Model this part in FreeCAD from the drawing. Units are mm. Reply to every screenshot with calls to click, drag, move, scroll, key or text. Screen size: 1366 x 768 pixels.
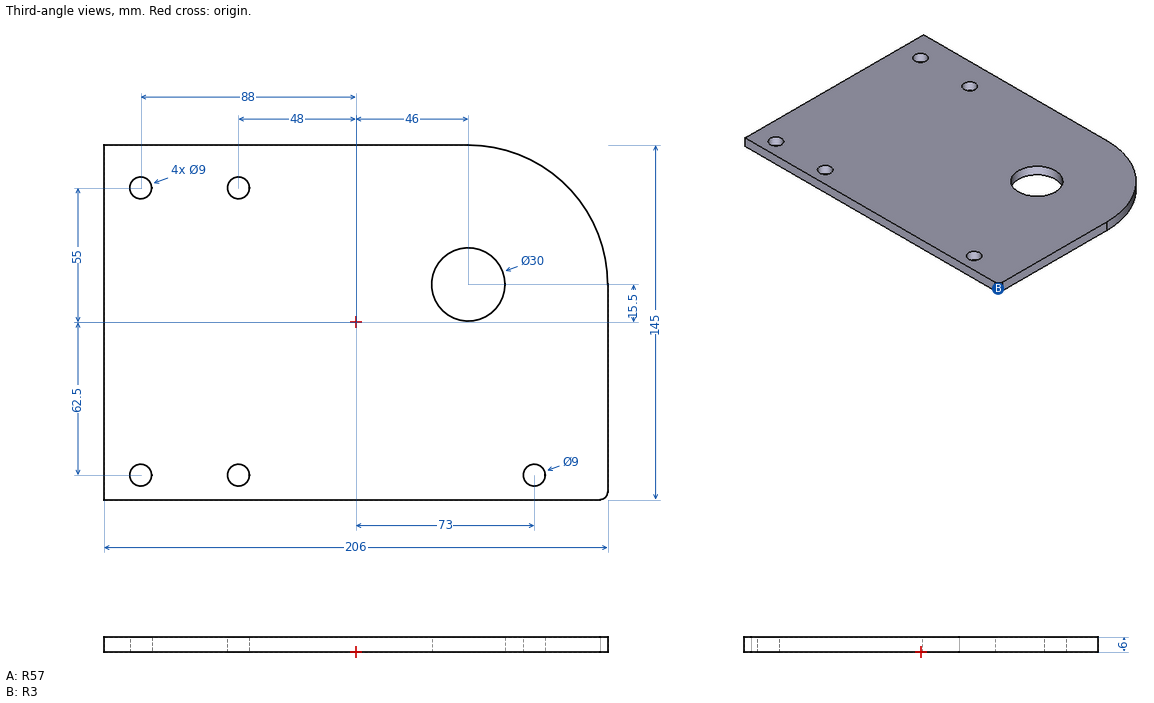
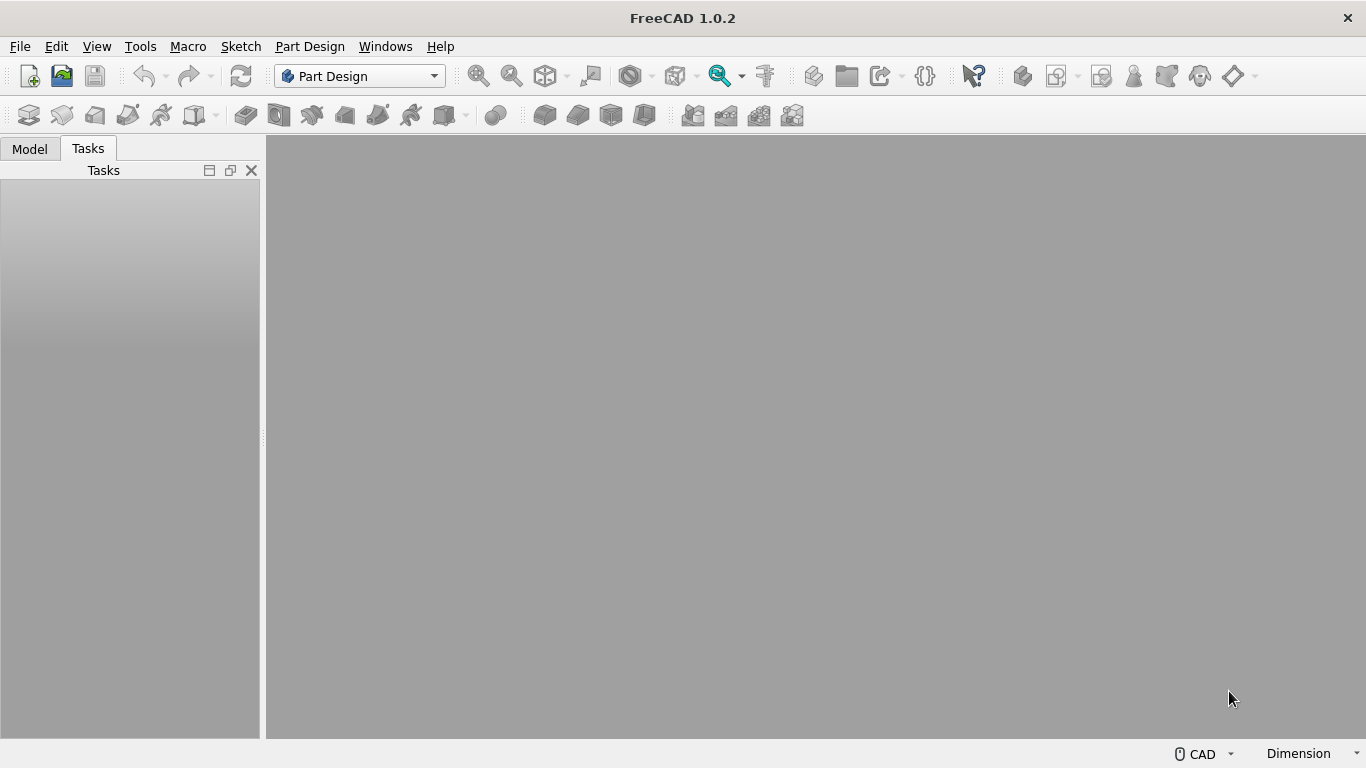
click(29, 76)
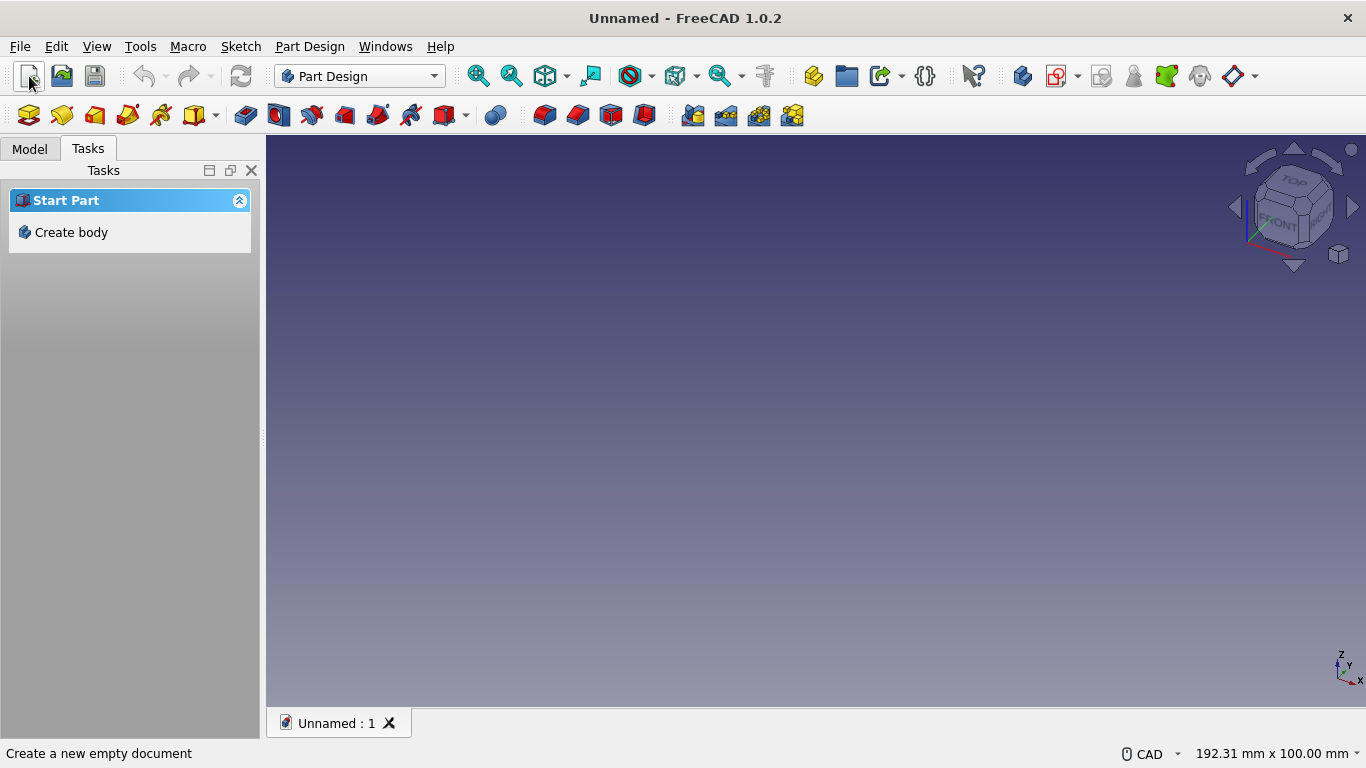
click(1056, 76)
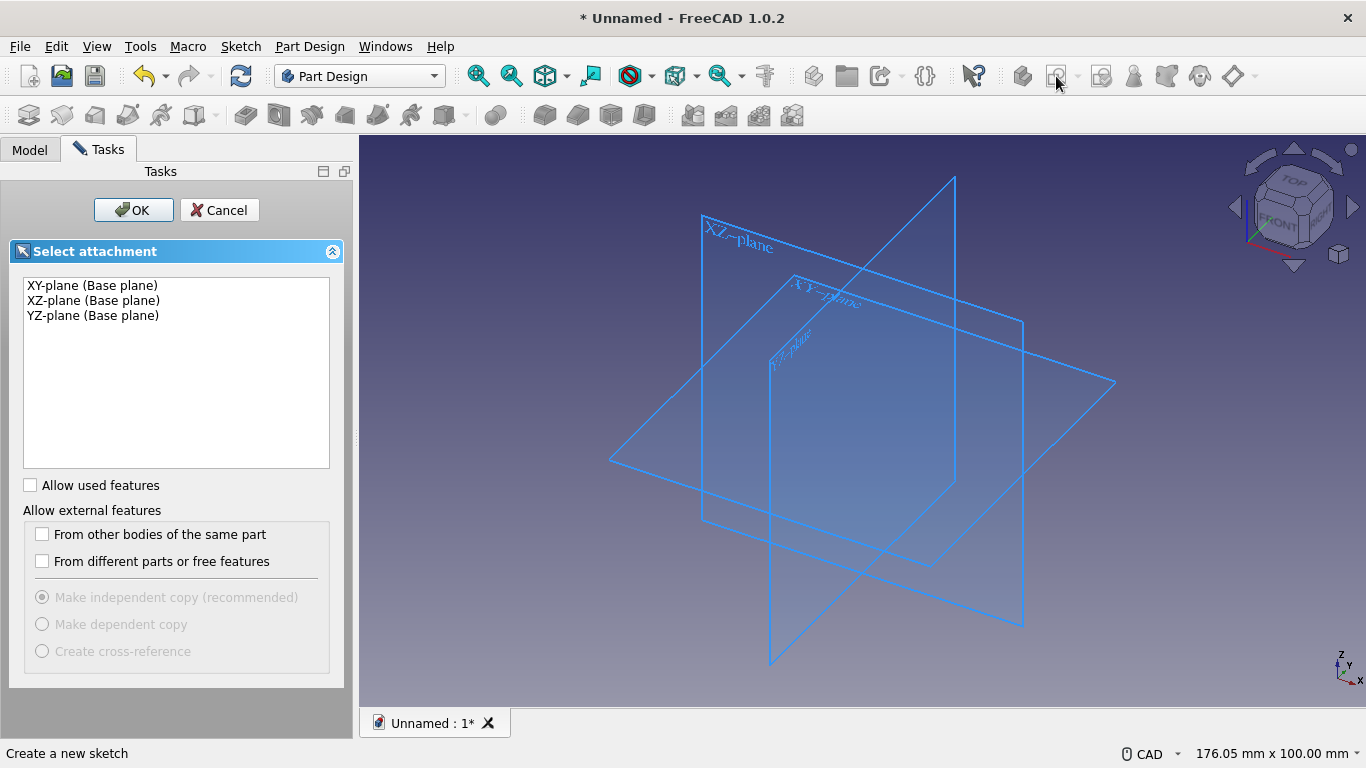
click(84, 286)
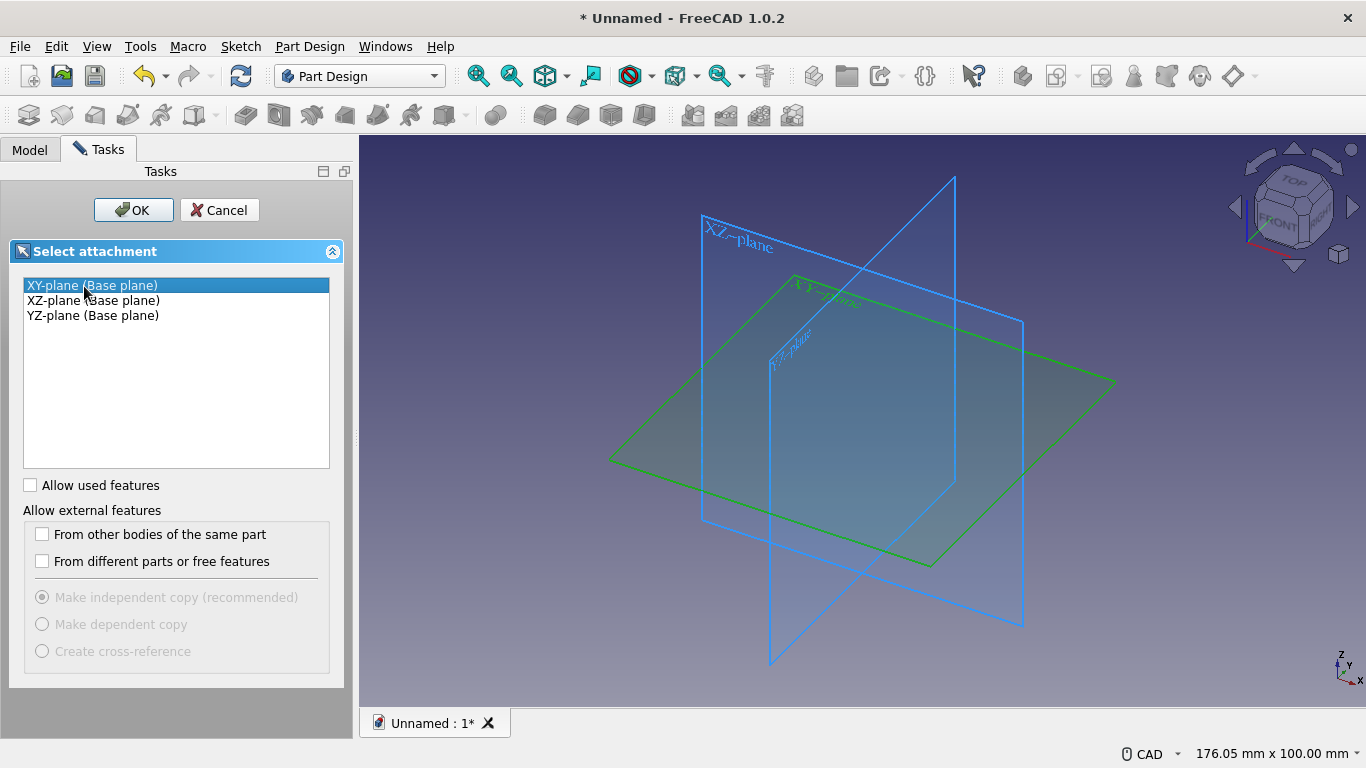
click(134, 210)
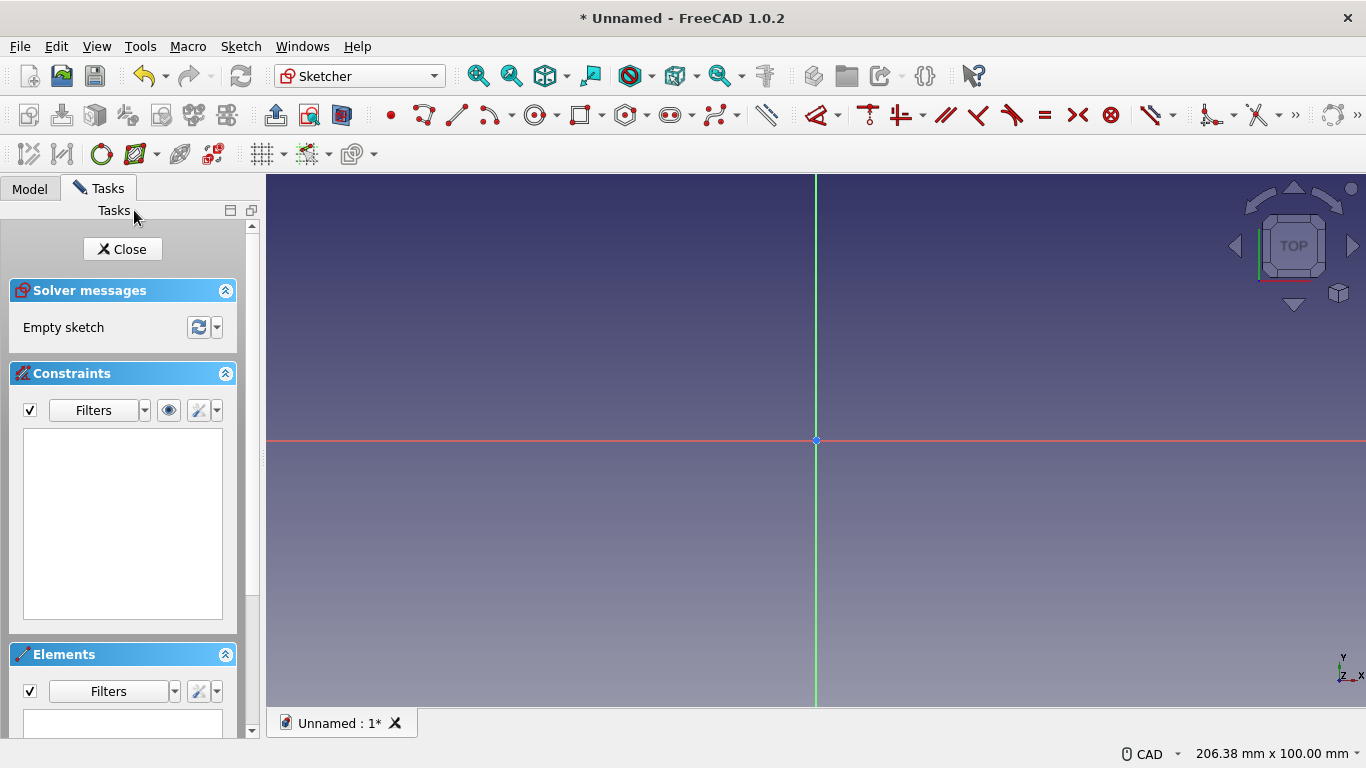
scroll(692, 440, down, 4)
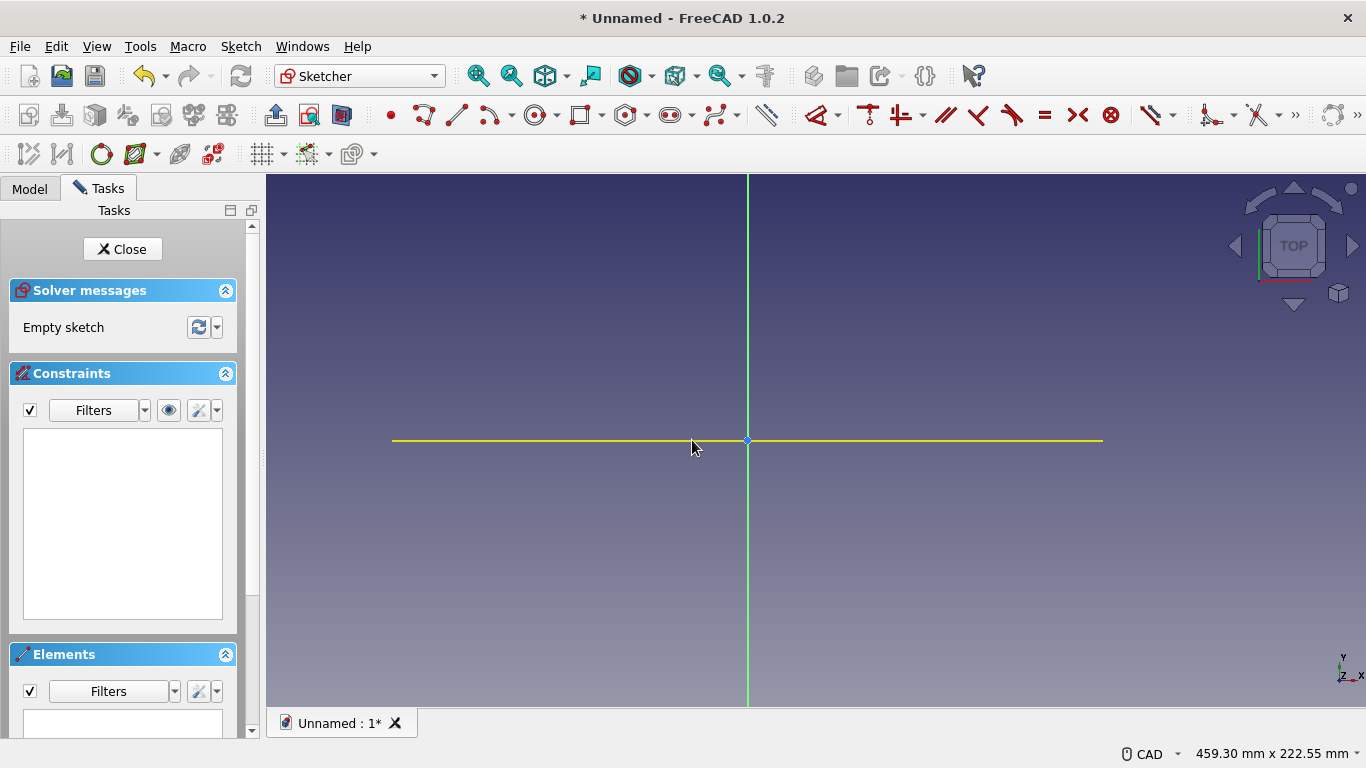
key(g)
key(v)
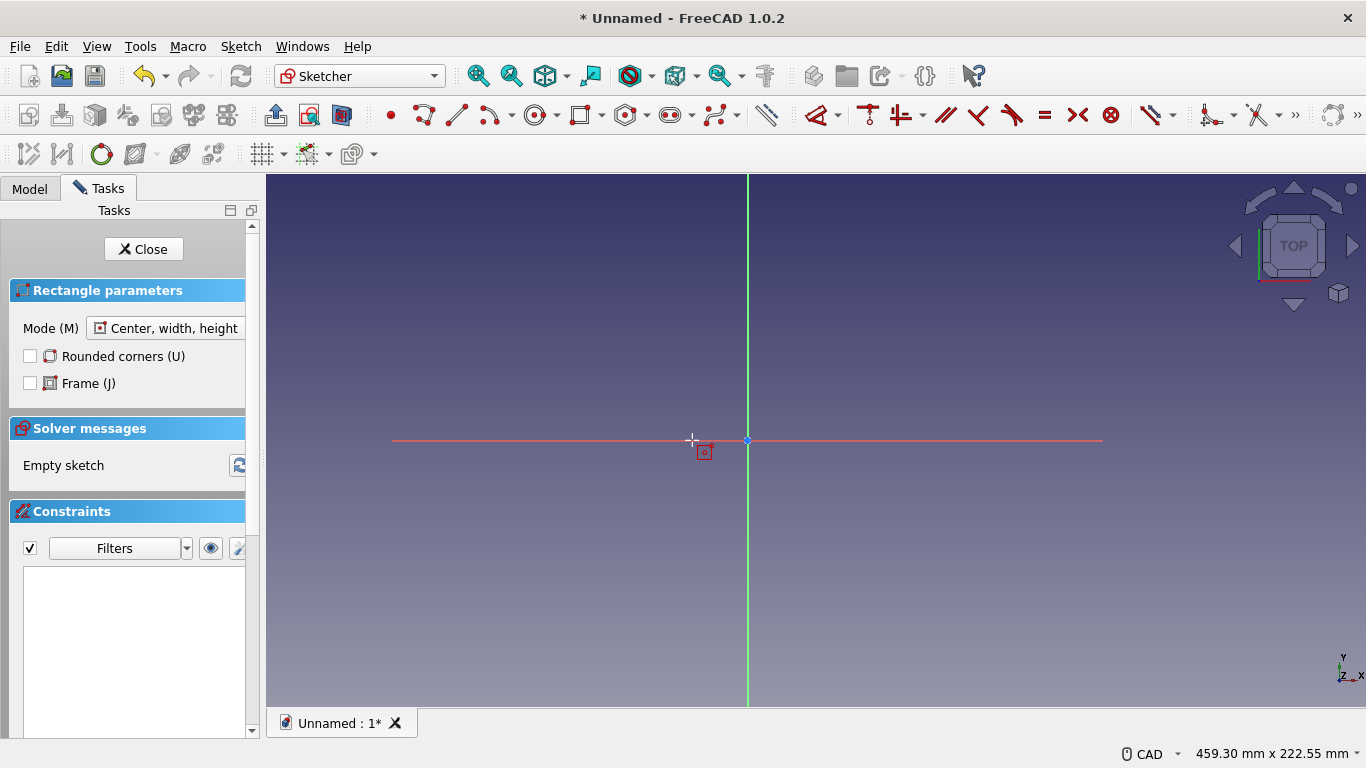
click(748, 440)
move(995, 267)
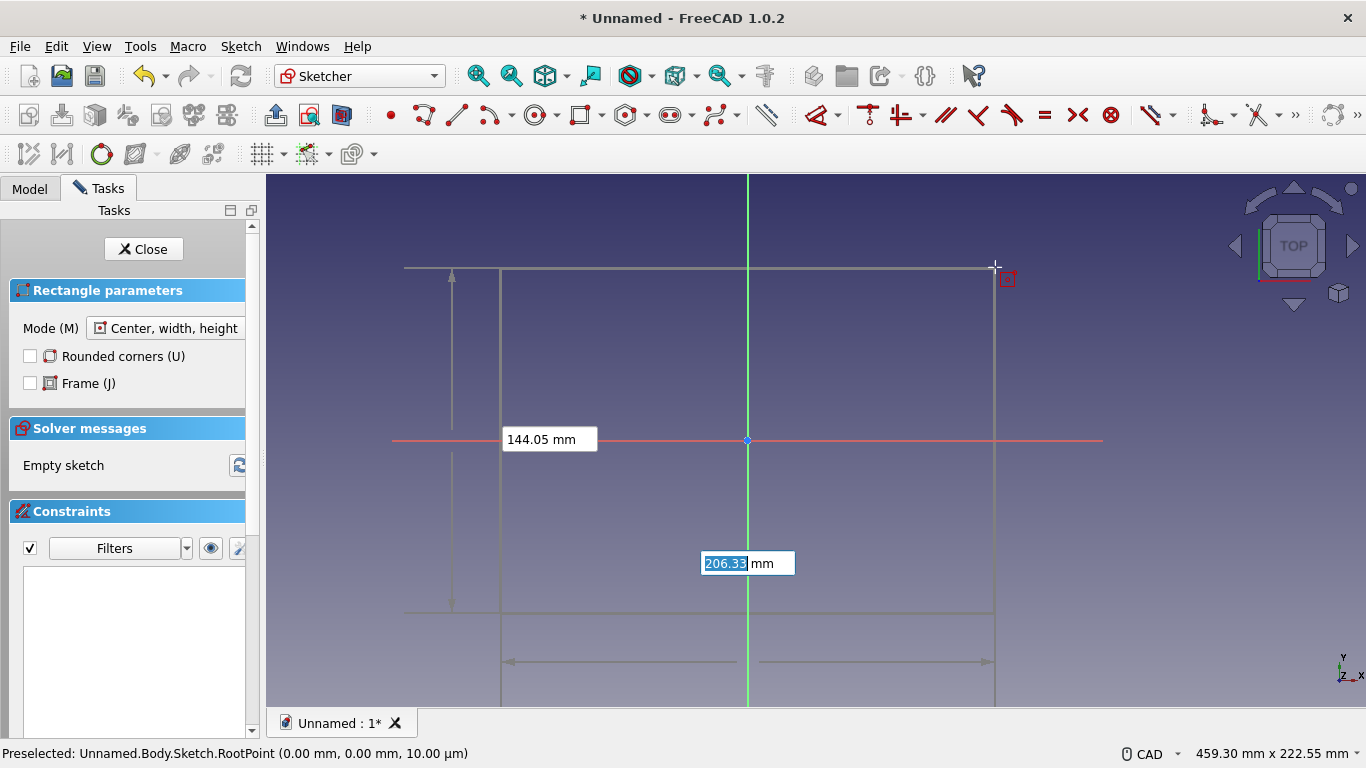
text(206)
key(Tab)
text(145)
key(Return)
key(Escape)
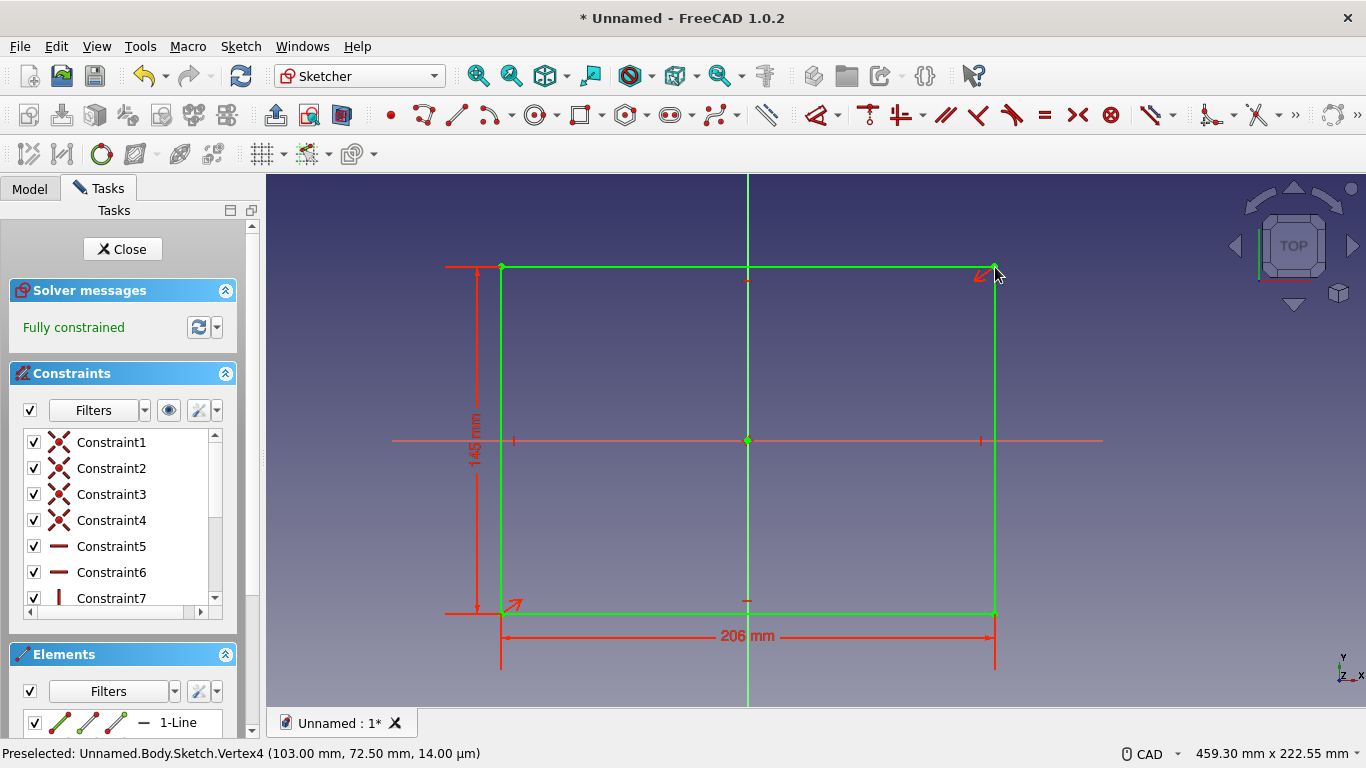
click(123, 249)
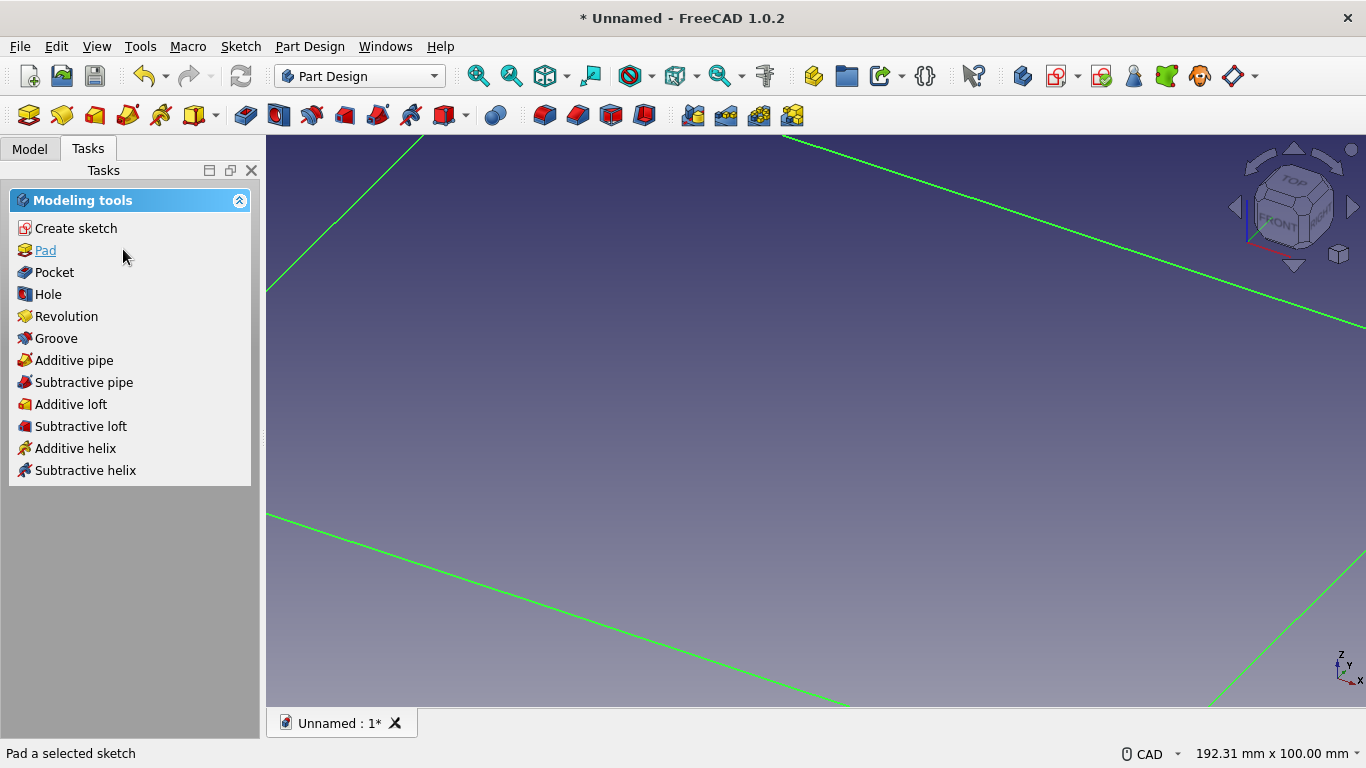
click(29, 116)